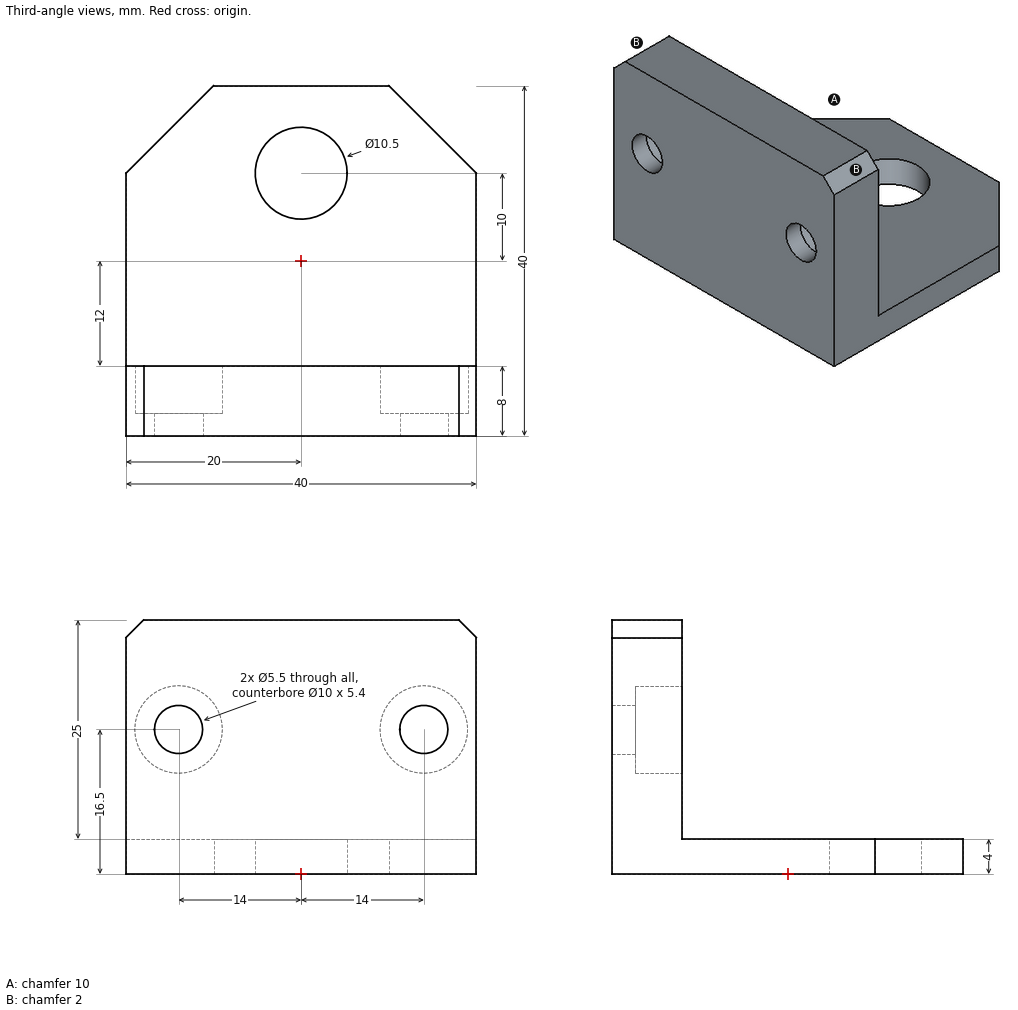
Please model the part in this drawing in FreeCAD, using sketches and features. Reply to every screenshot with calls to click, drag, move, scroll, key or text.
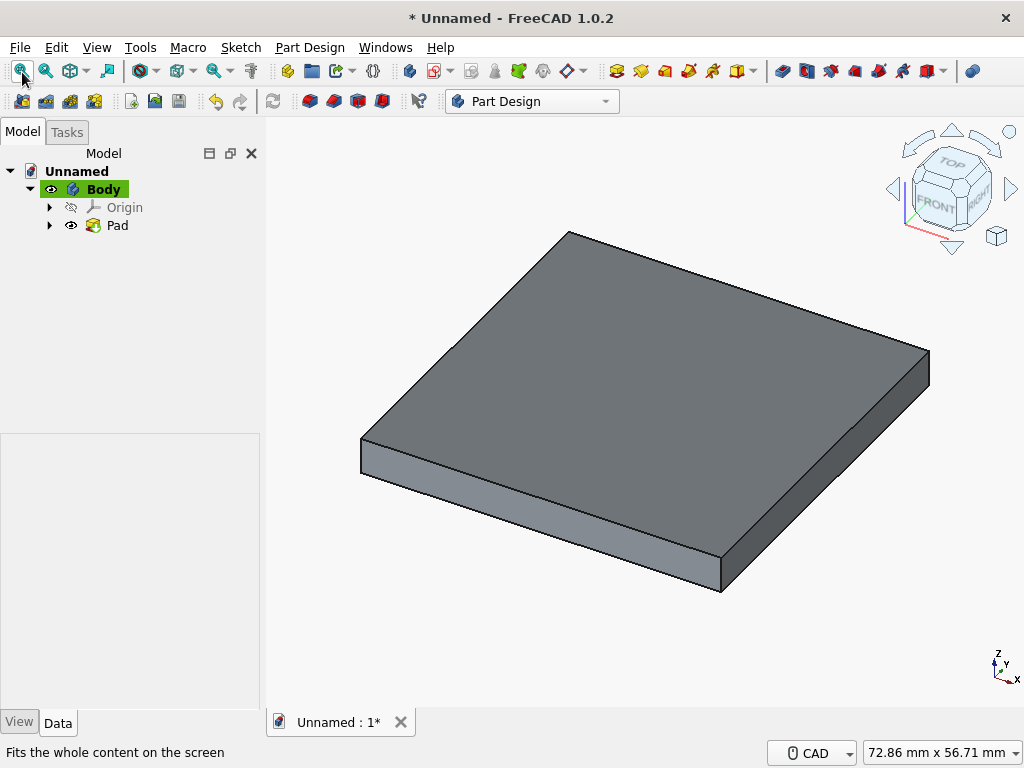
click(645, 394)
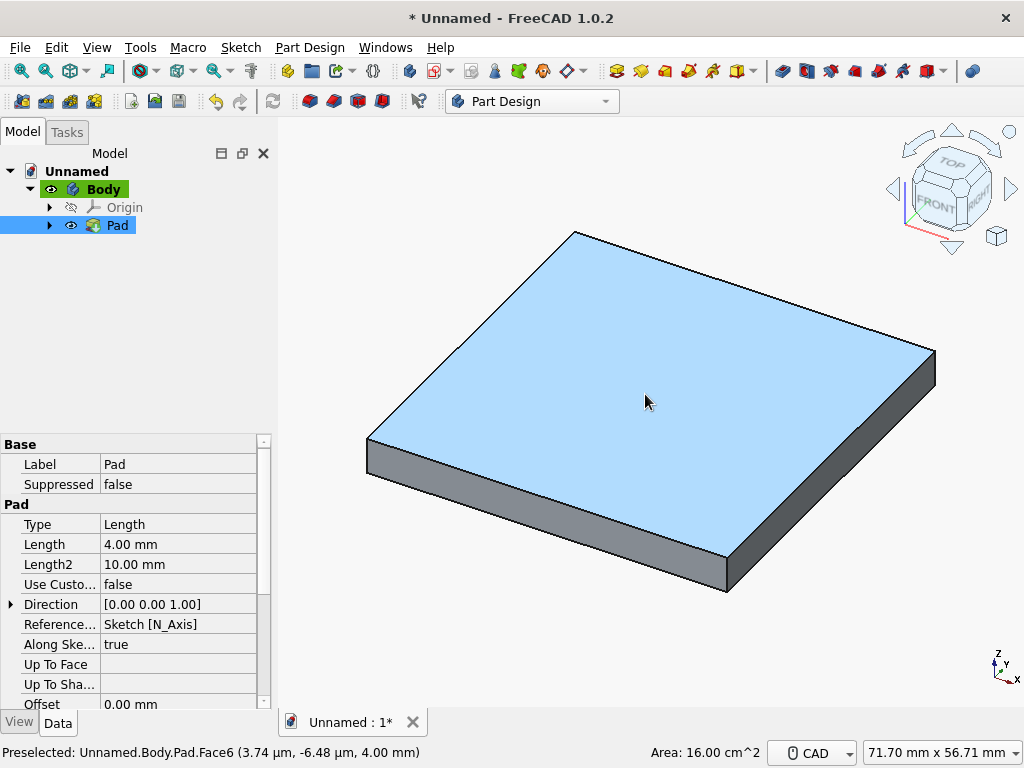
click(434, 72)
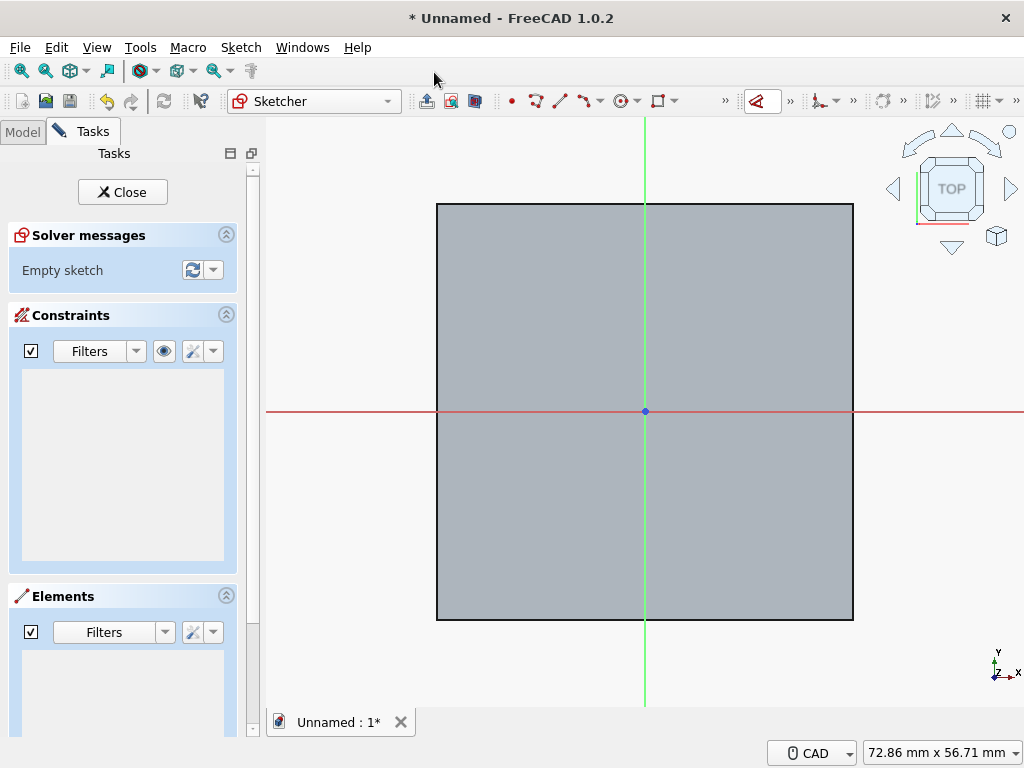
scroll(294, 145, down, 1)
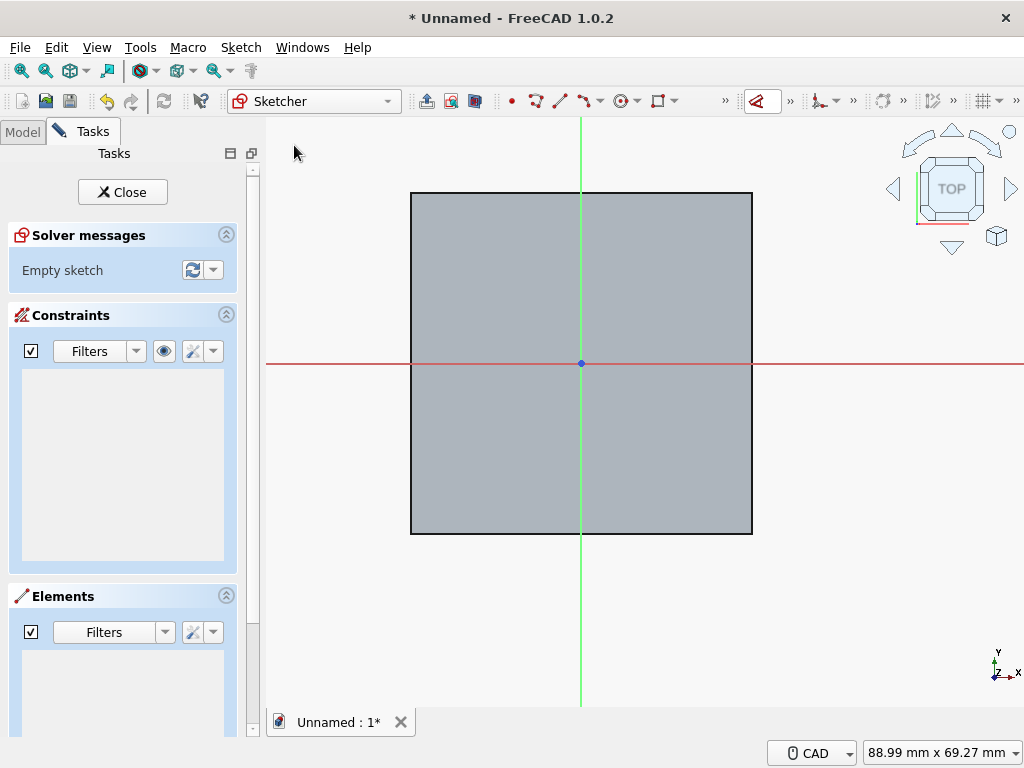
click(658, 102)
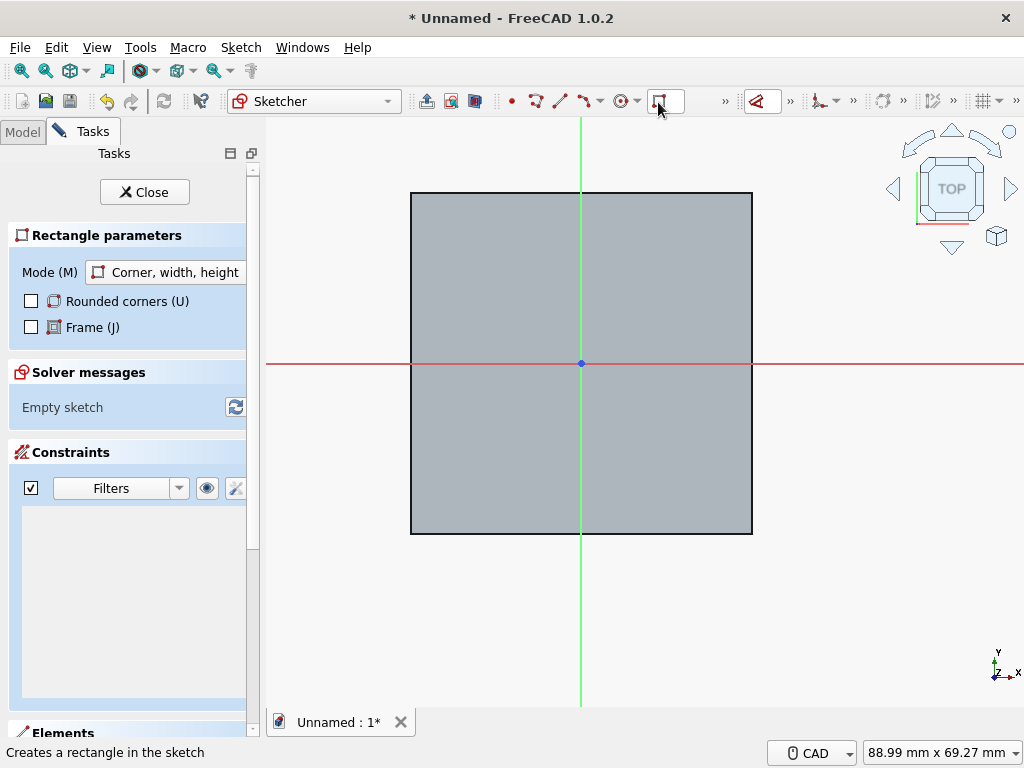
click(411, 466)
move(752, 534)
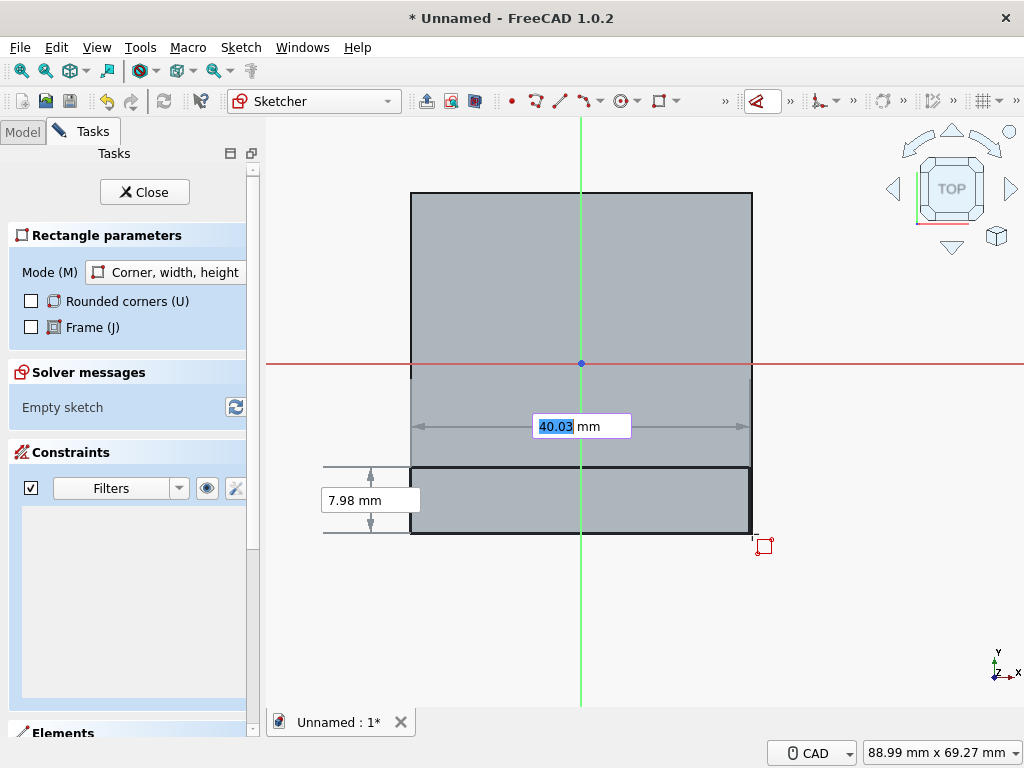
text(40)
key(Tab)
text(8)
key(Return)
key(Escape)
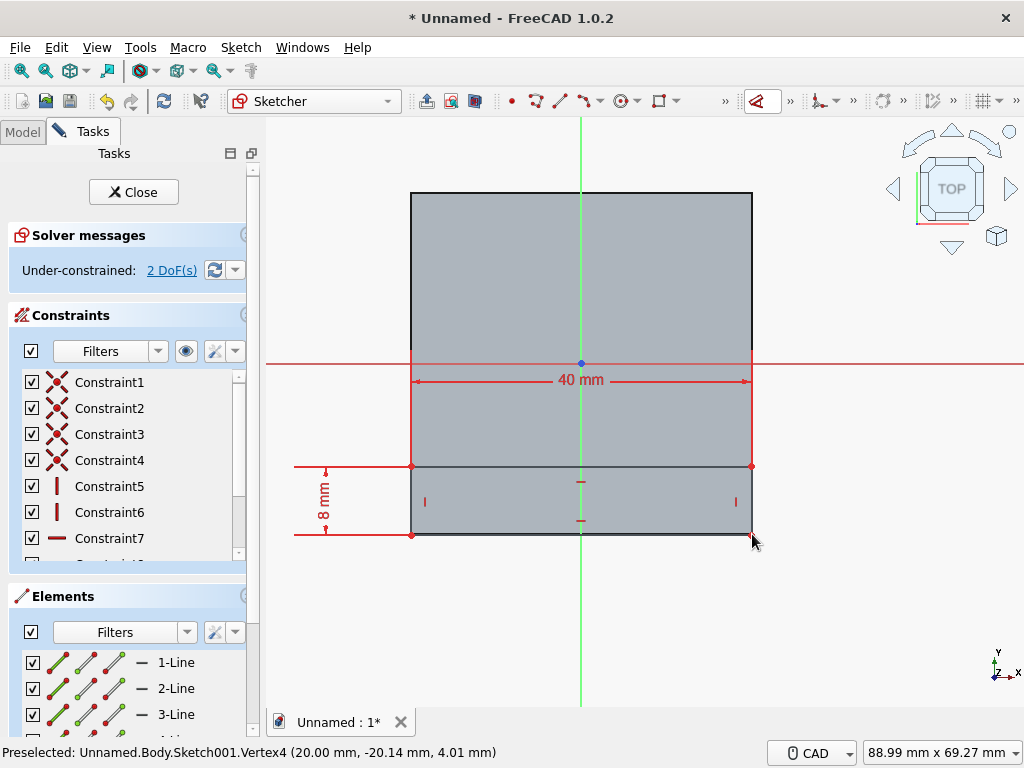
click(756, 102)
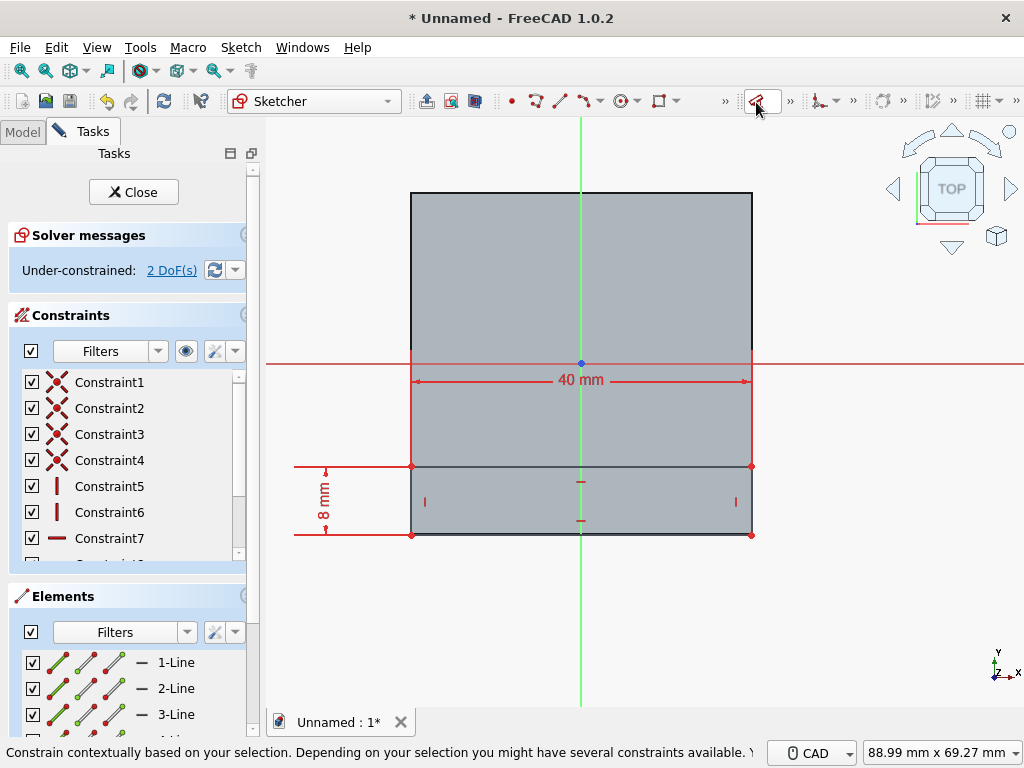
click(411, 467)
click(496, 330)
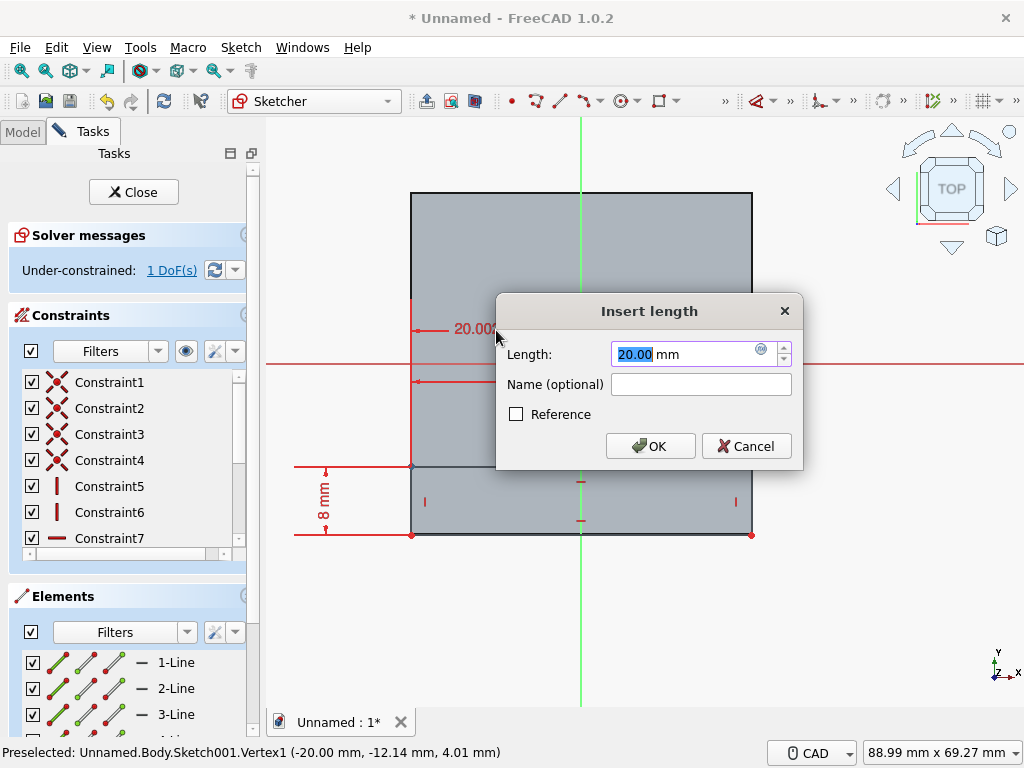
text(20)
key(Return)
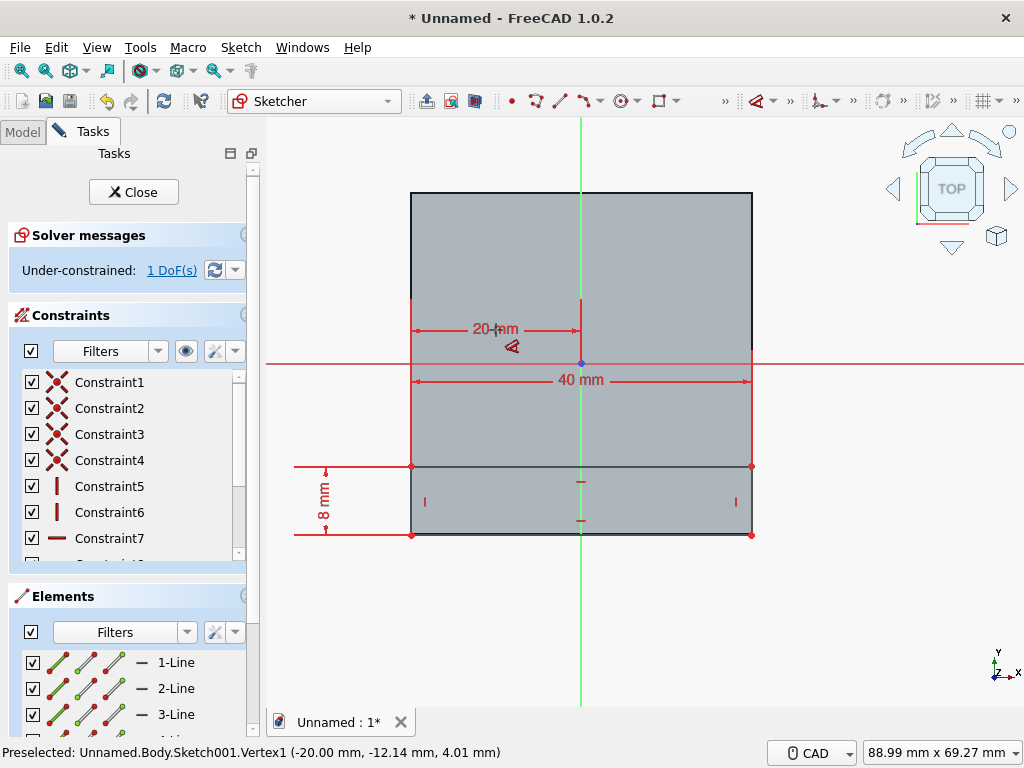
click(411, 467)
click(377, 415)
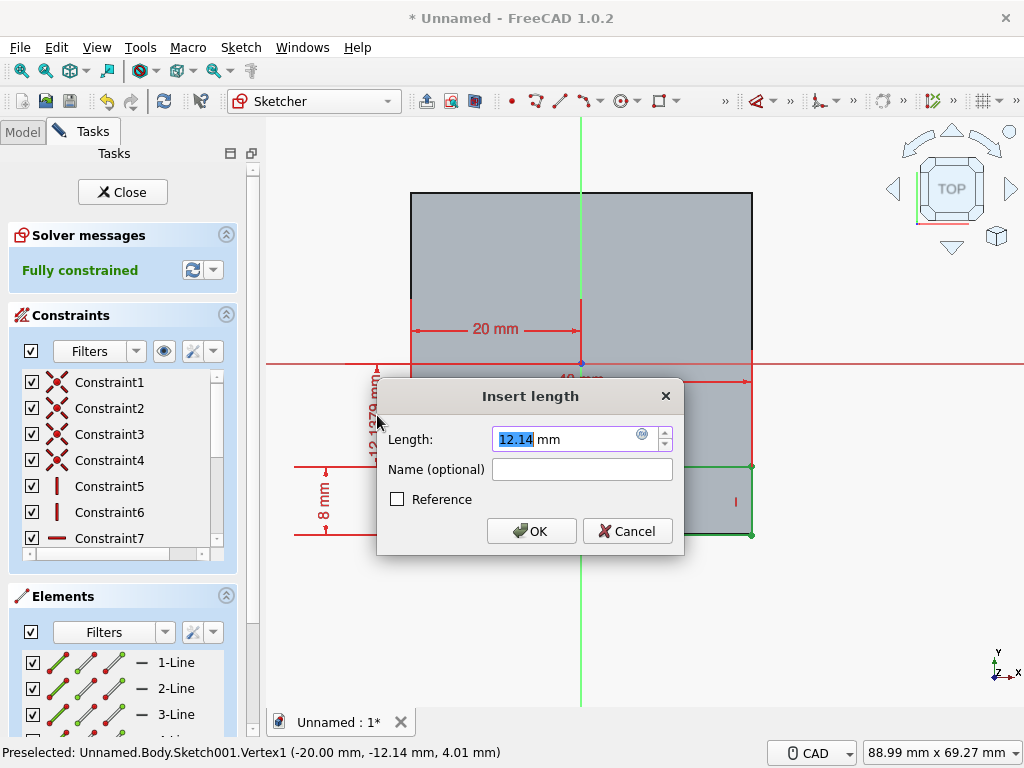
text(12)
key(Return)
key(Escape)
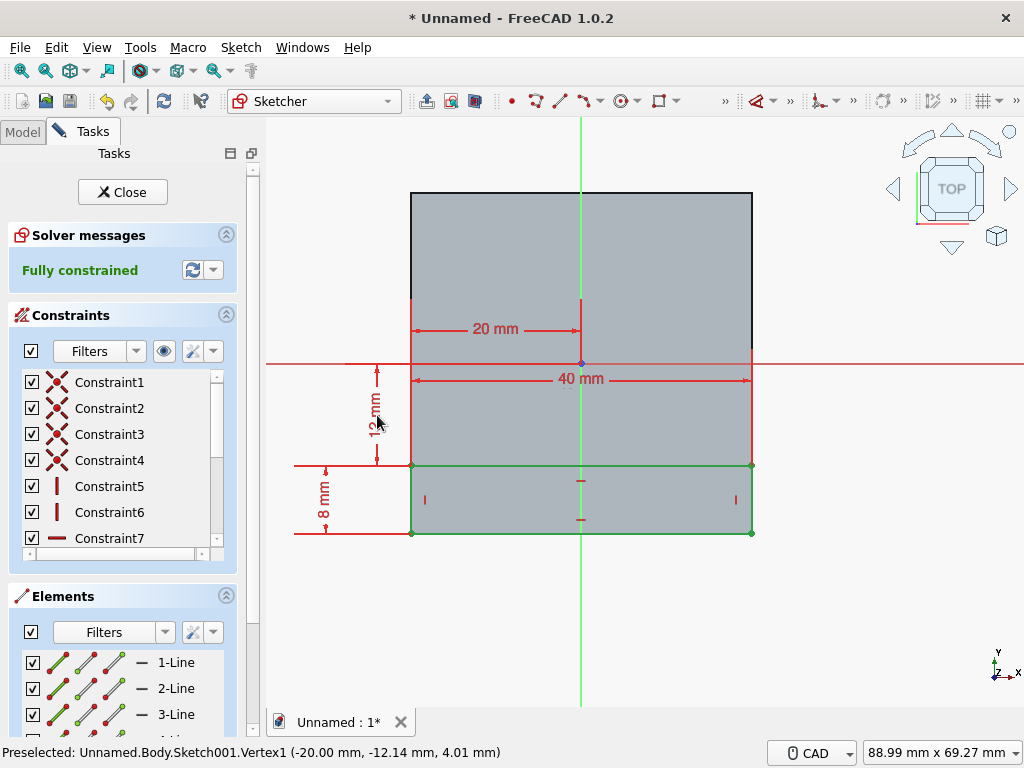
click(123, 192)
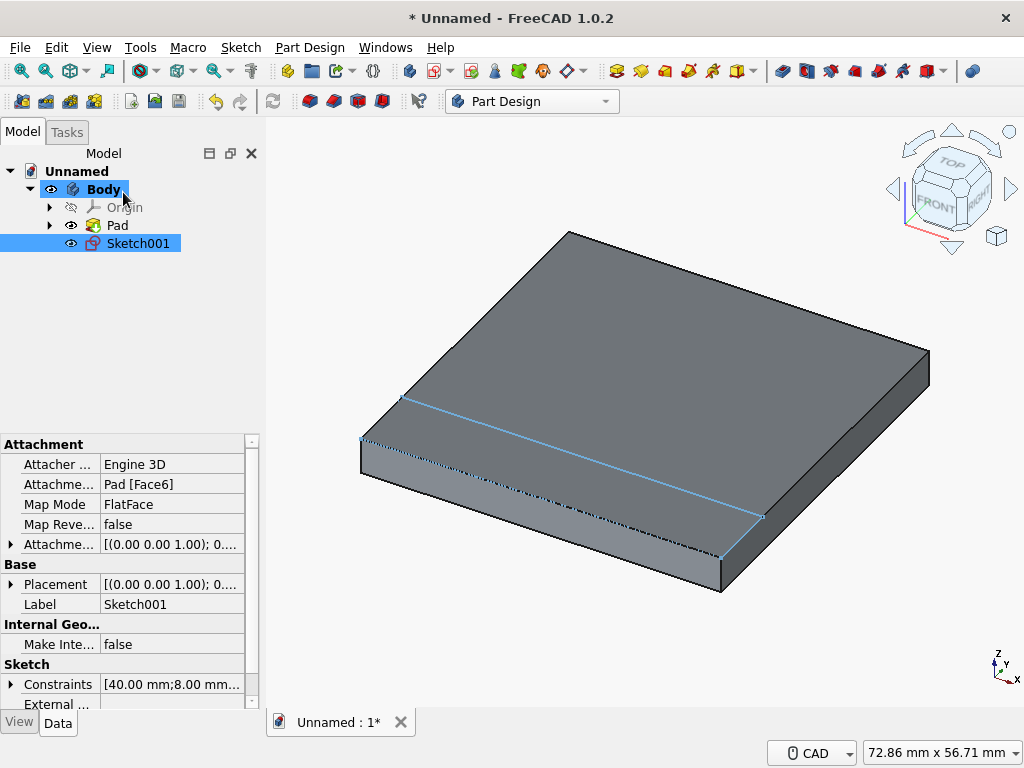
click(618, 72)